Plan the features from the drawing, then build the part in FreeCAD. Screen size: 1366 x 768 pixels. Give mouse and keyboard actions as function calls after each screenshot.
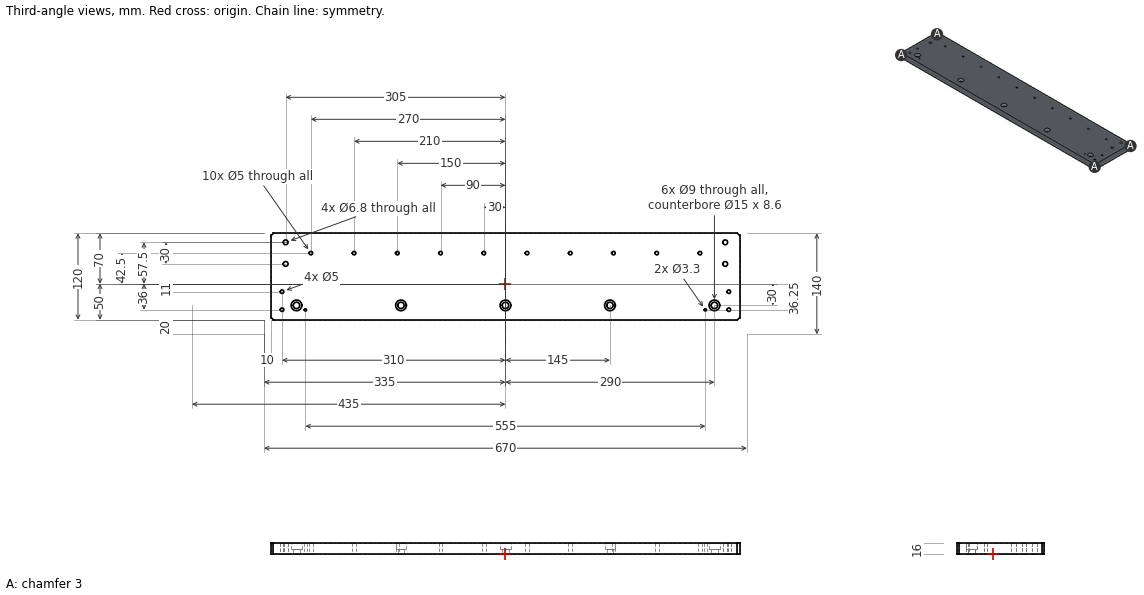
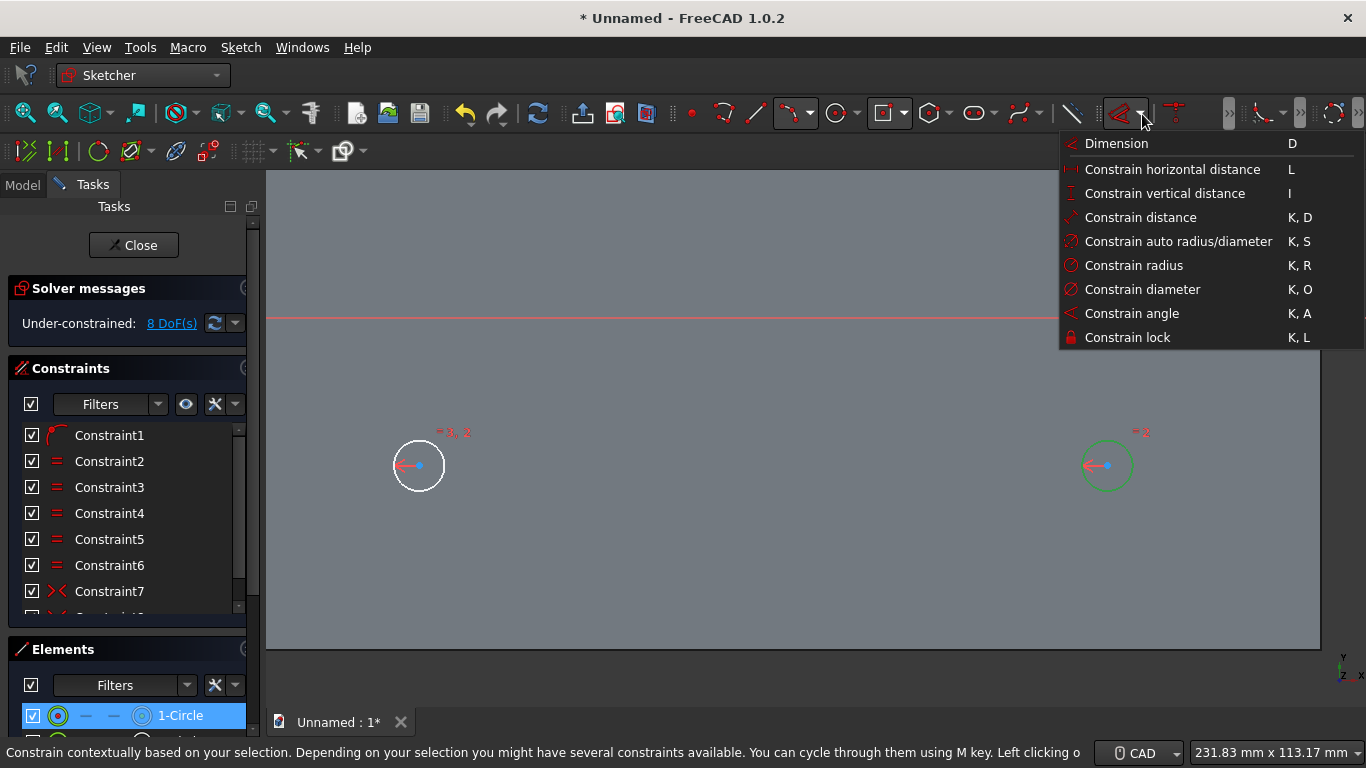
click(1212, 289)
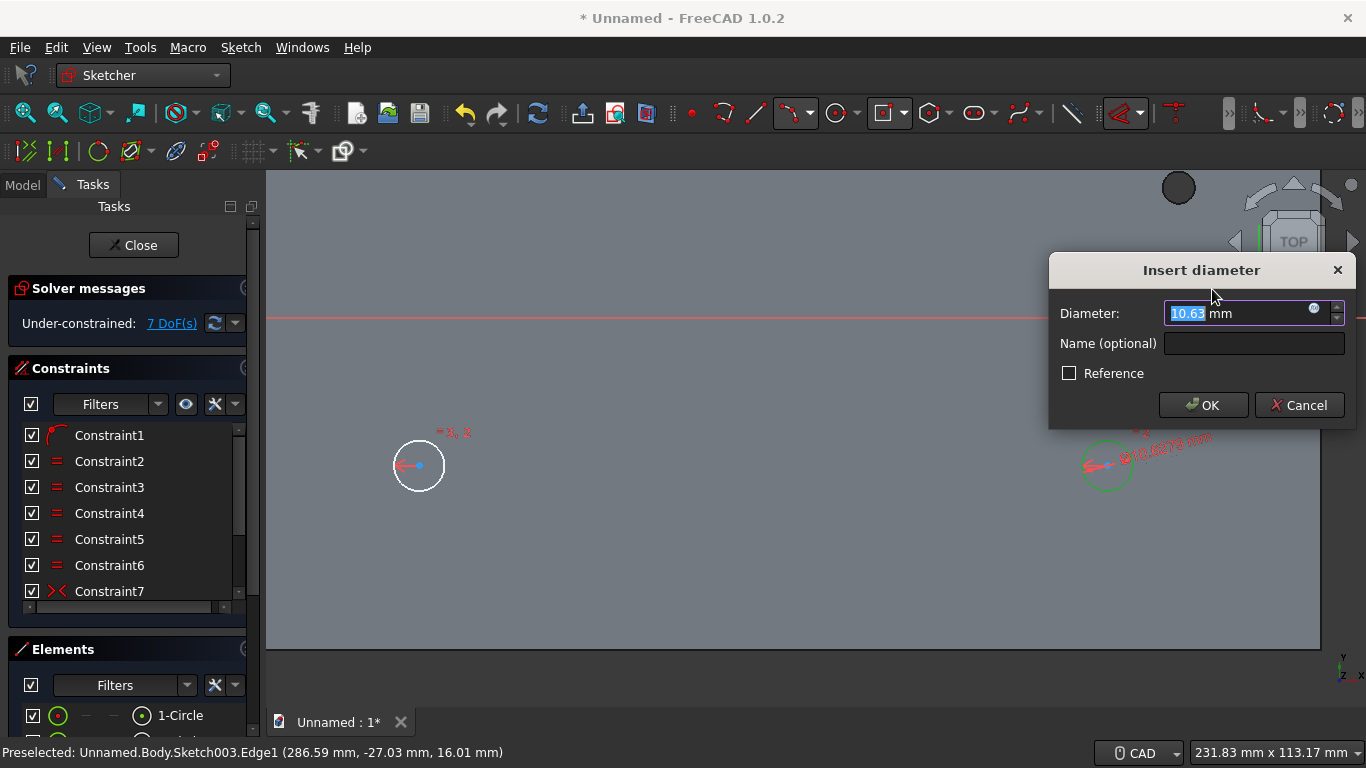
text(9)
key(Return)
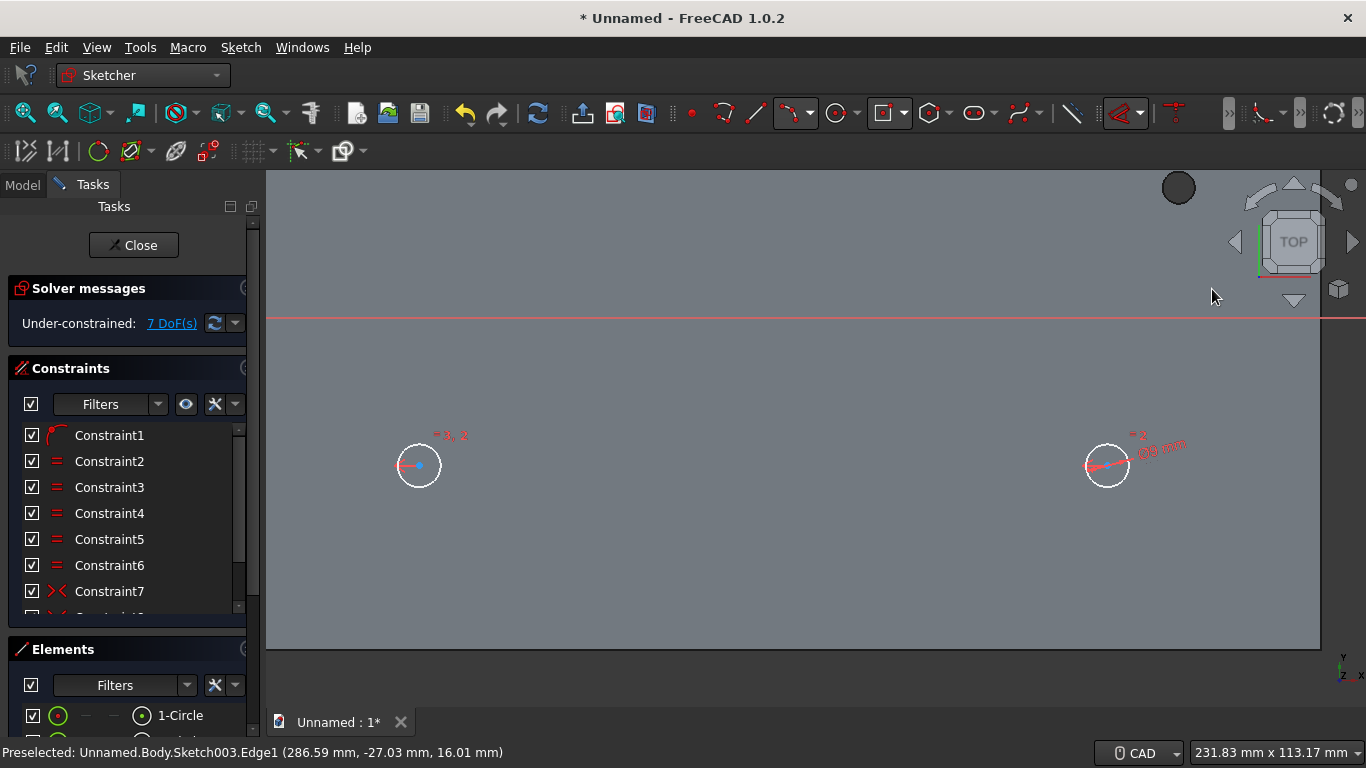
scroll(1092, 448, down, 8)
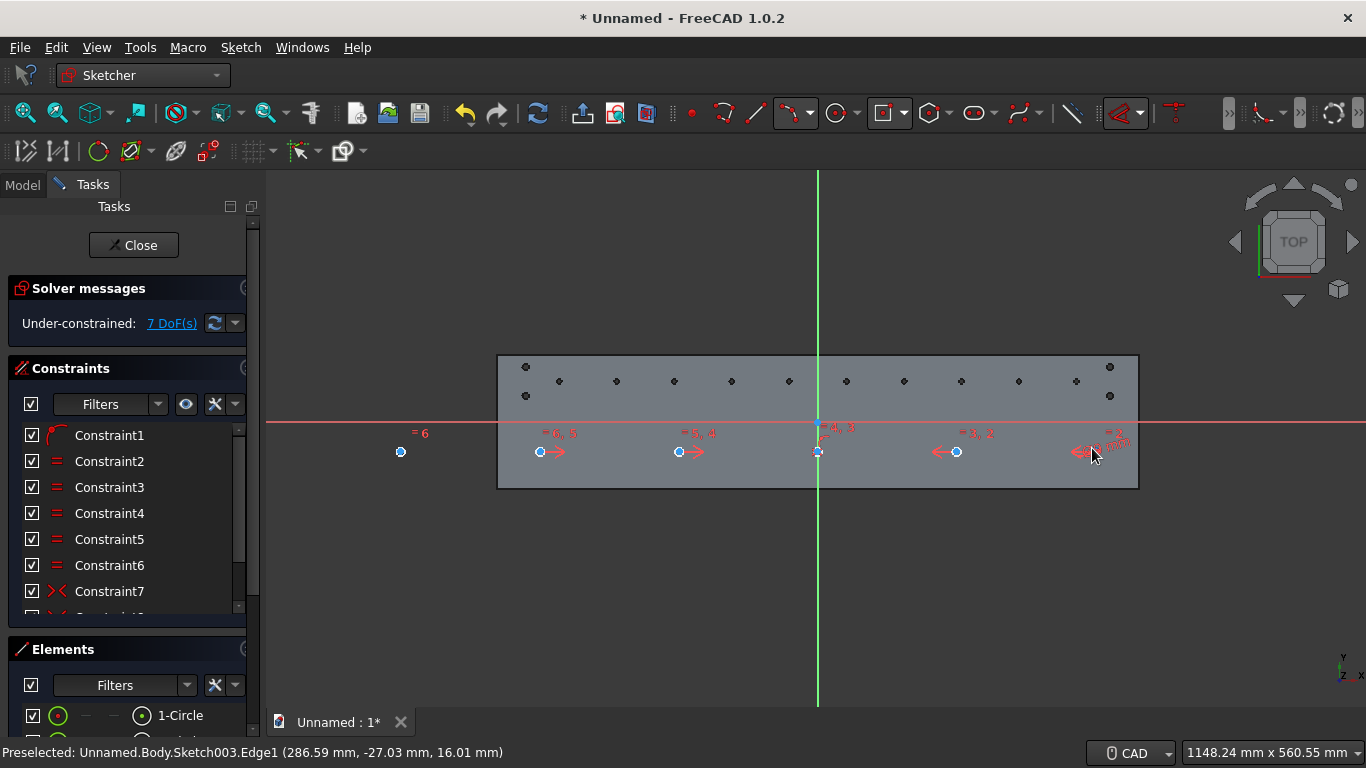
scroll(1096, 452, up, 2)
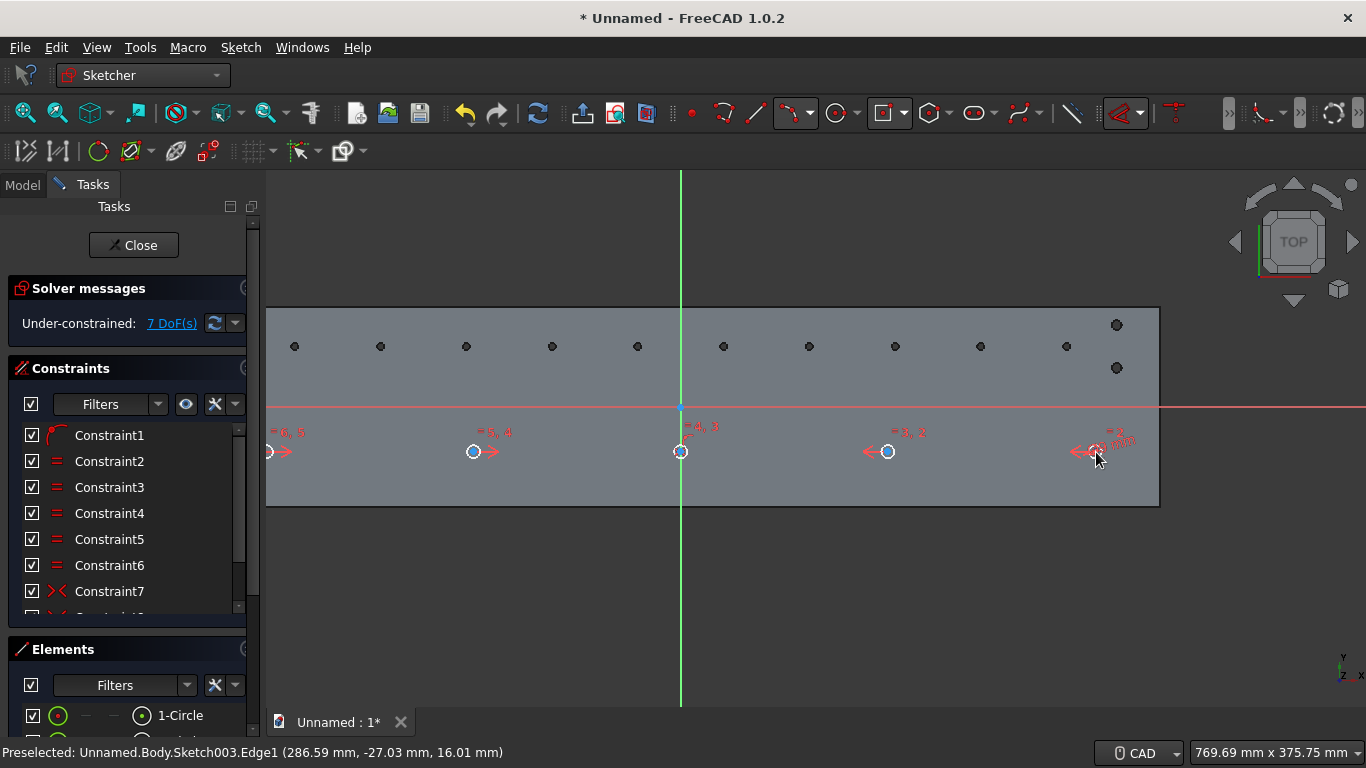
click(1095, 452)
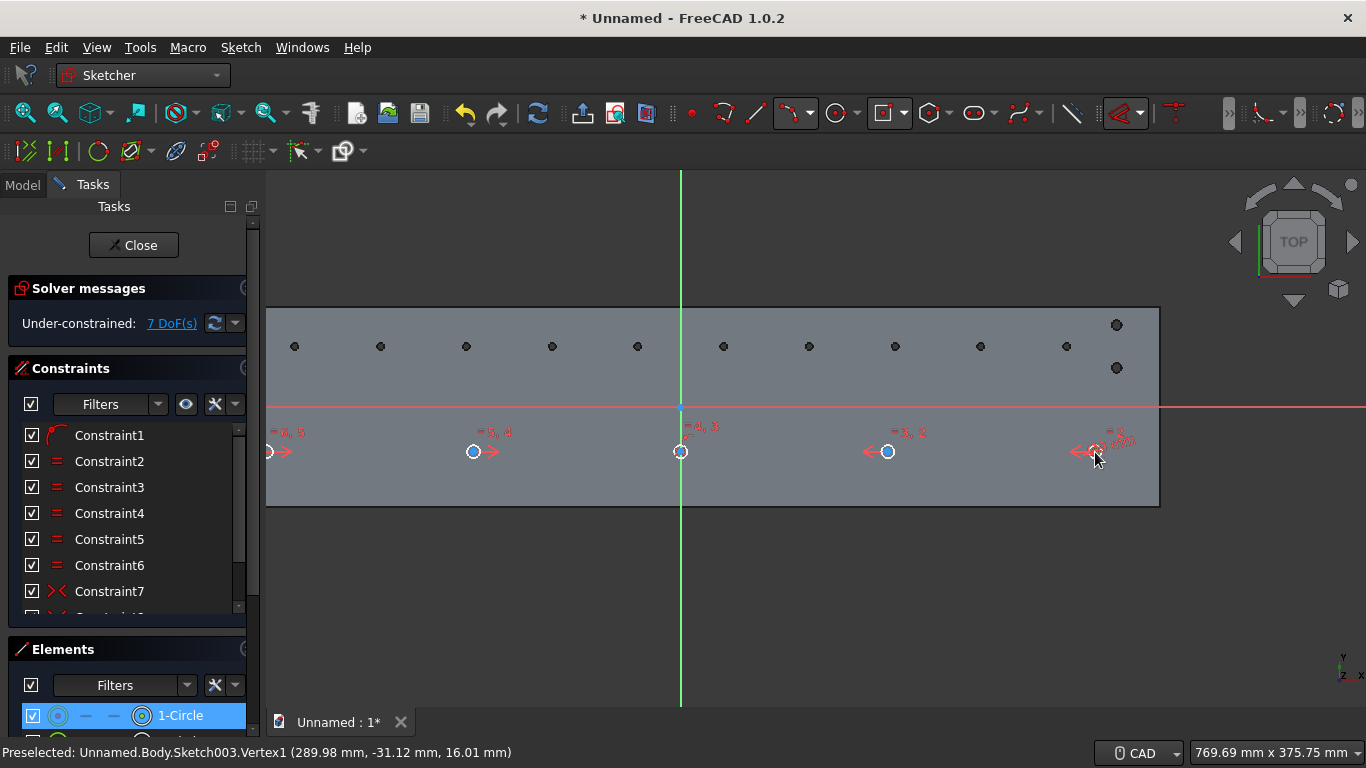
click(1142, 114)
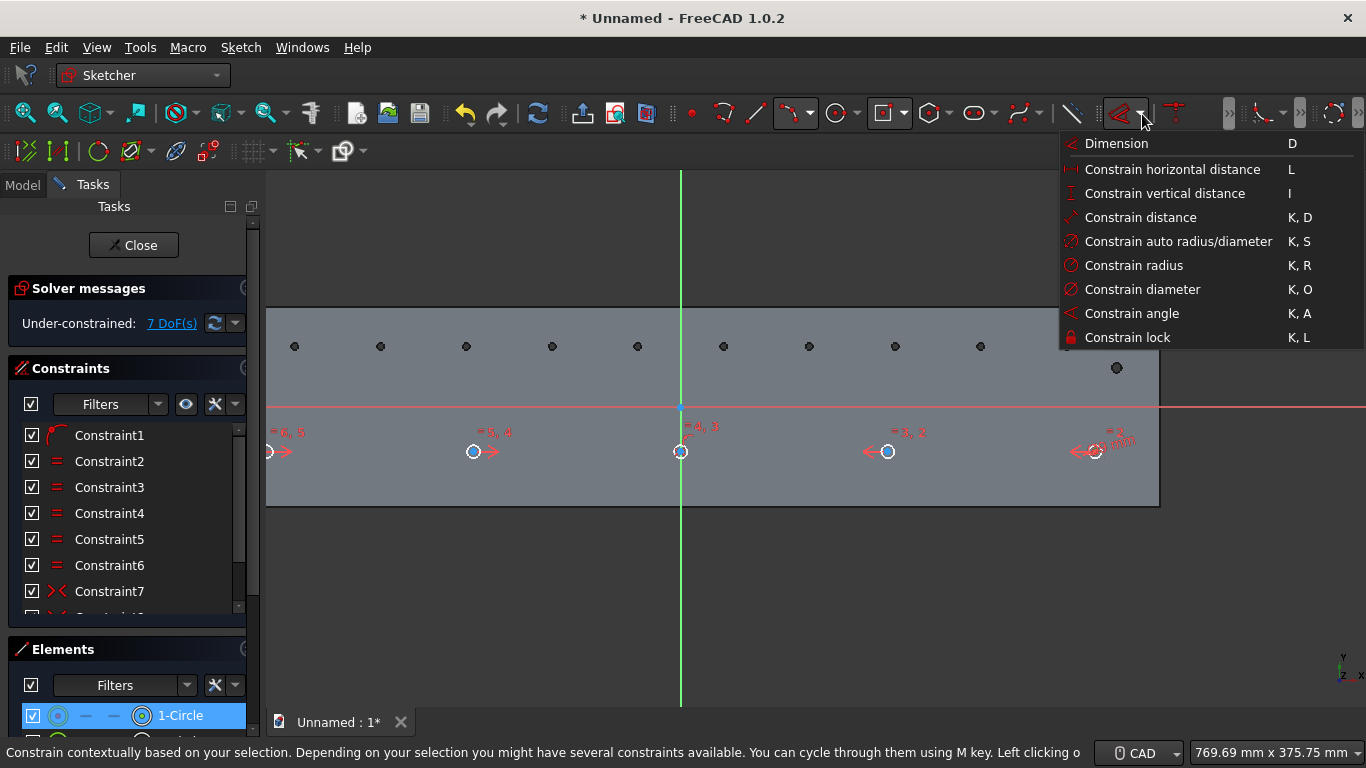
click(1212, 193)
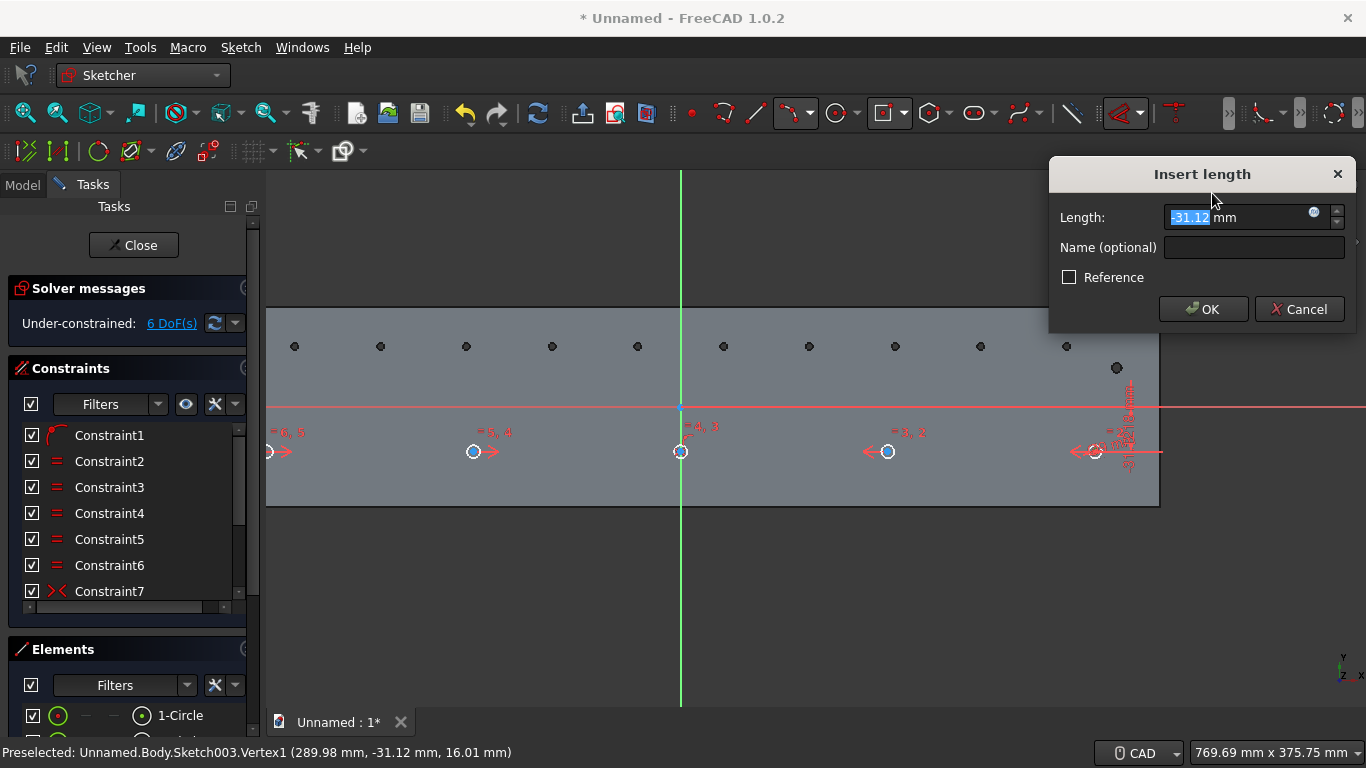
text(-30)
key(Return)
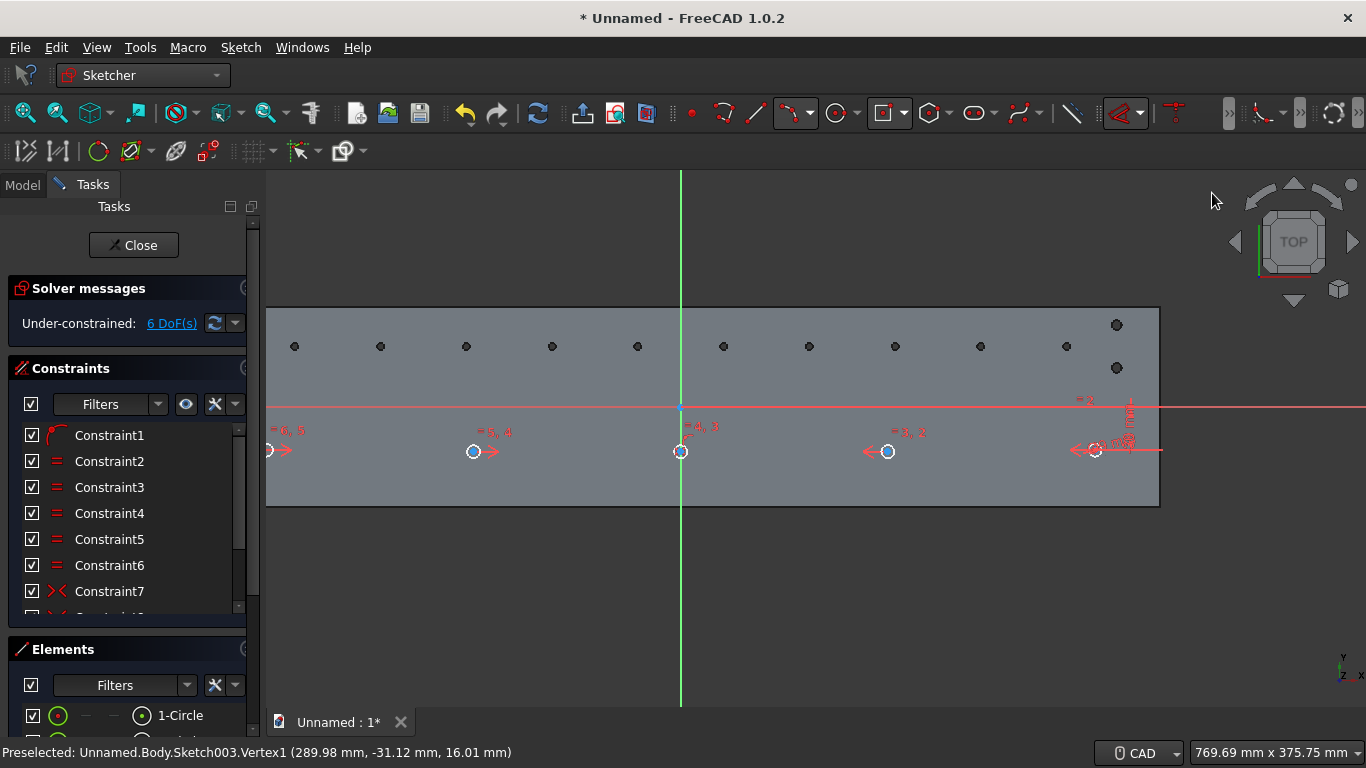
click(888, 452)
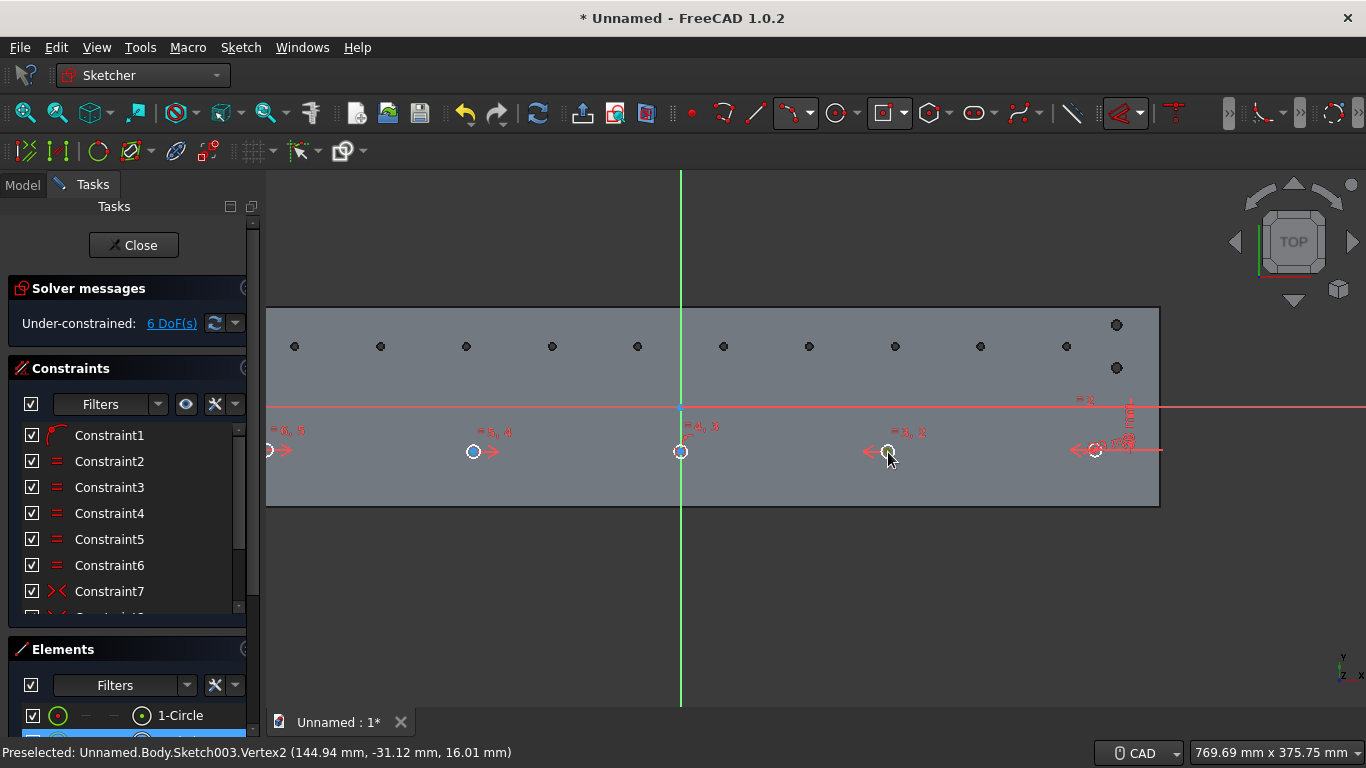
key(i)